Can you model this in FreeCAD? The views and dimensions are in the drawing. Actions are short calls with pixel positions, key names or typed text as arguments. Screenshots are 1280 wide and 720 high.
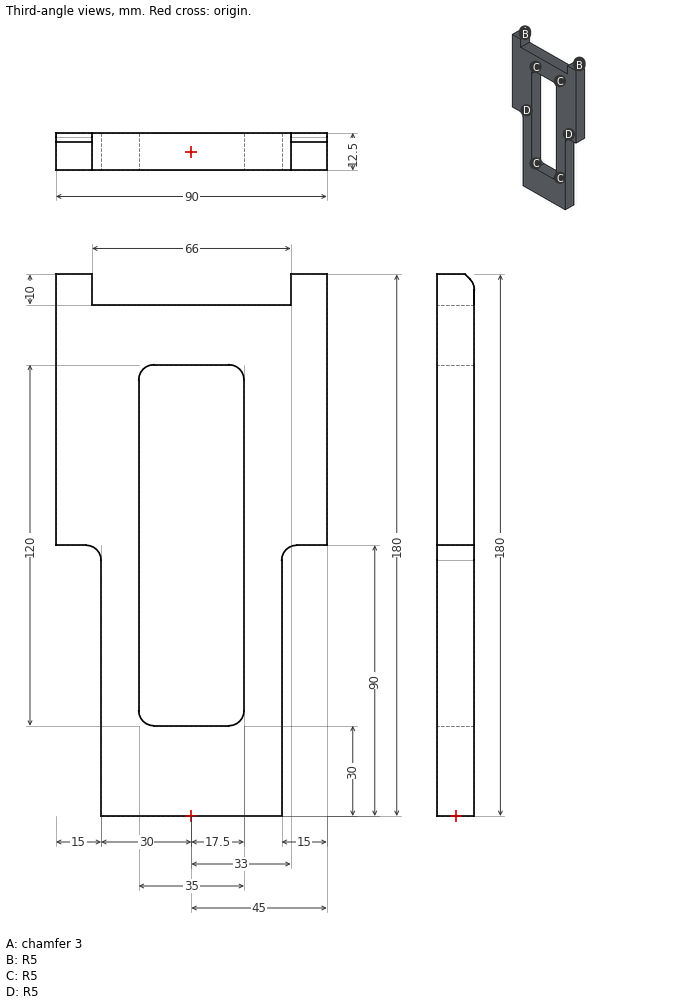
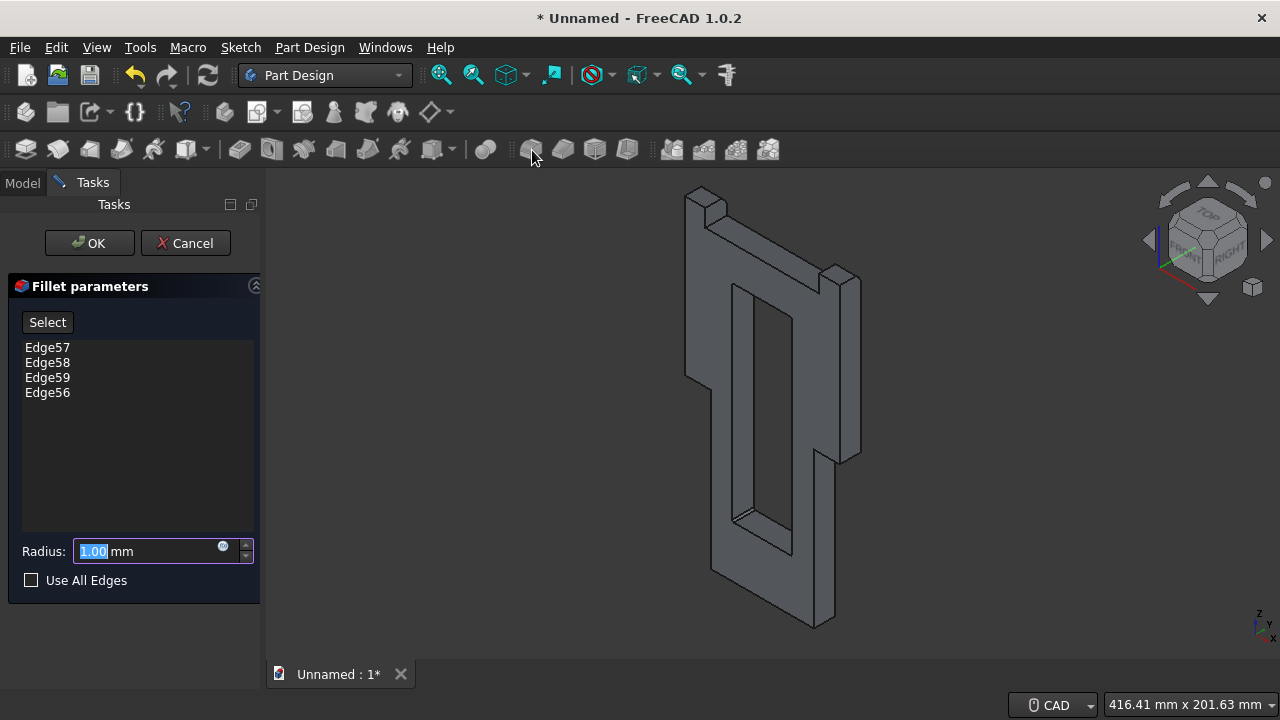
text(5)
key(Tab)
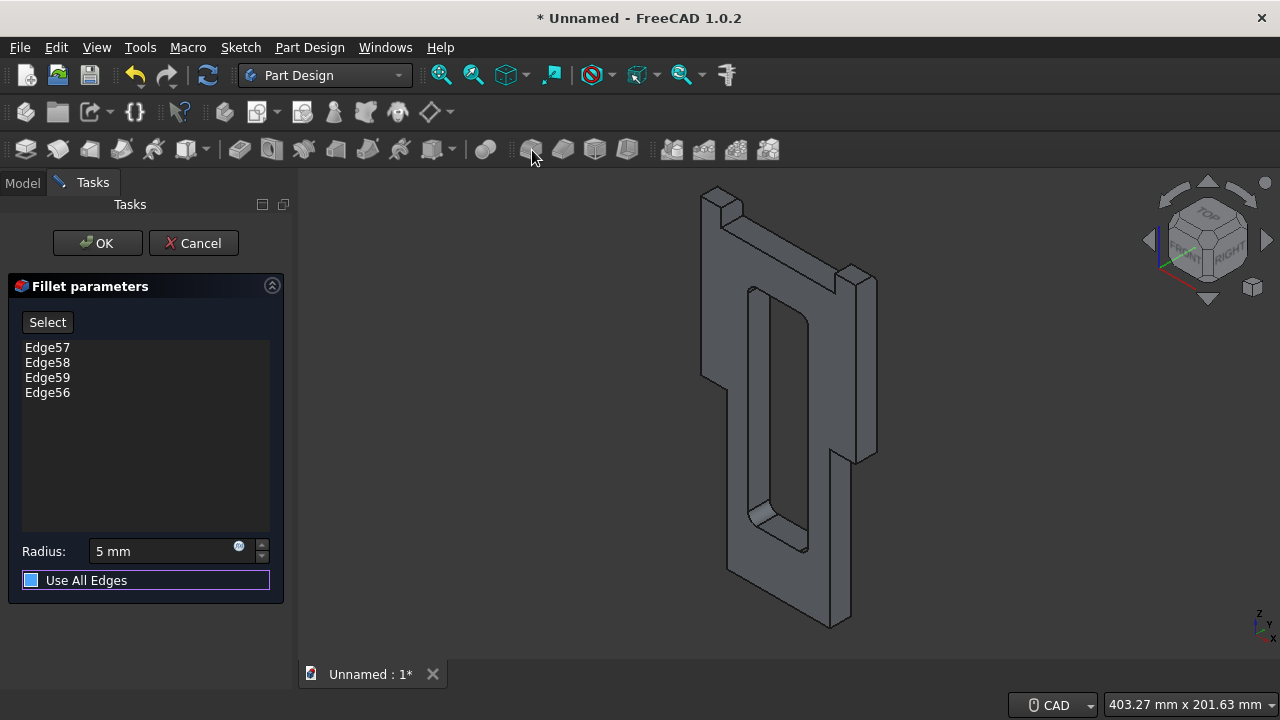
click(98, 243)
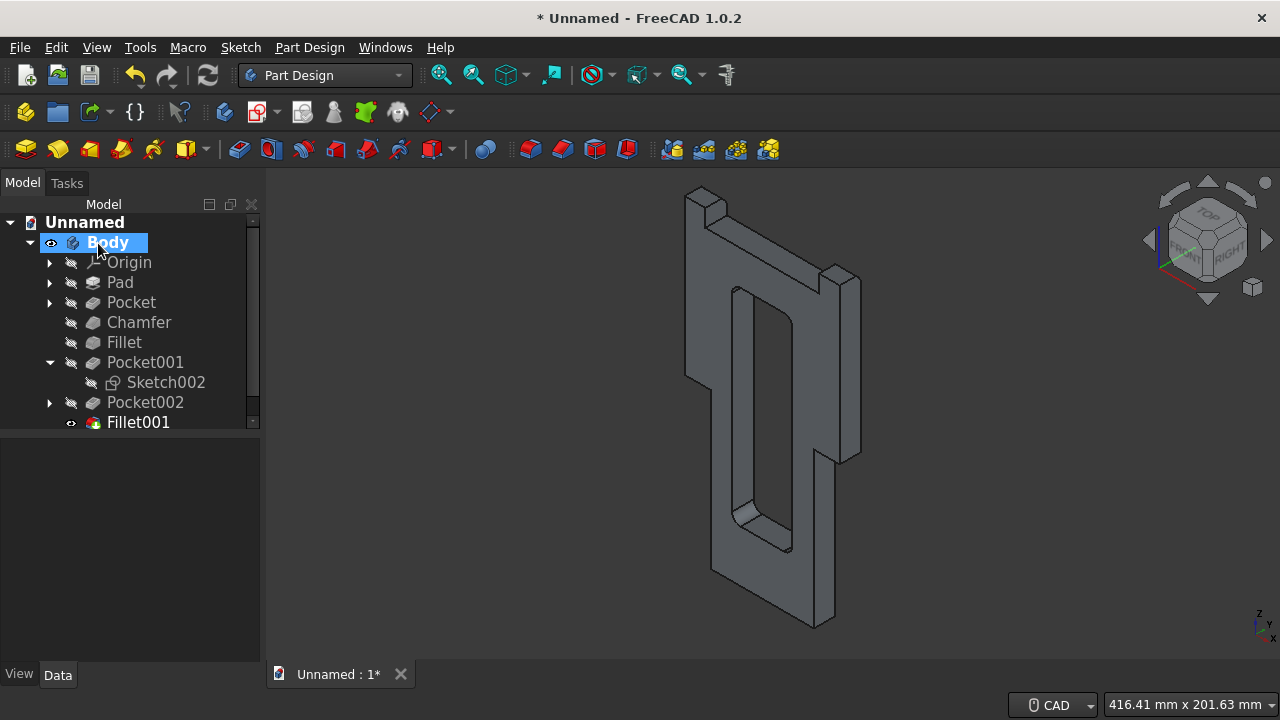
key(2)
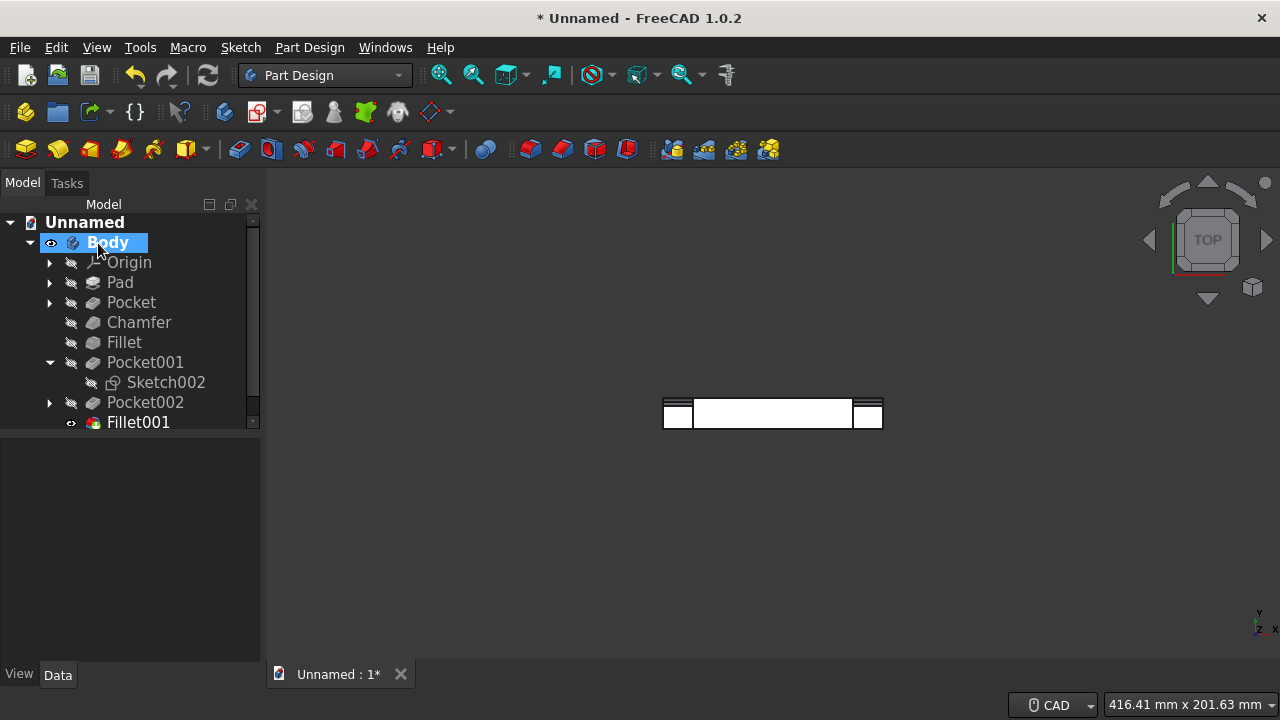
click(442, 76)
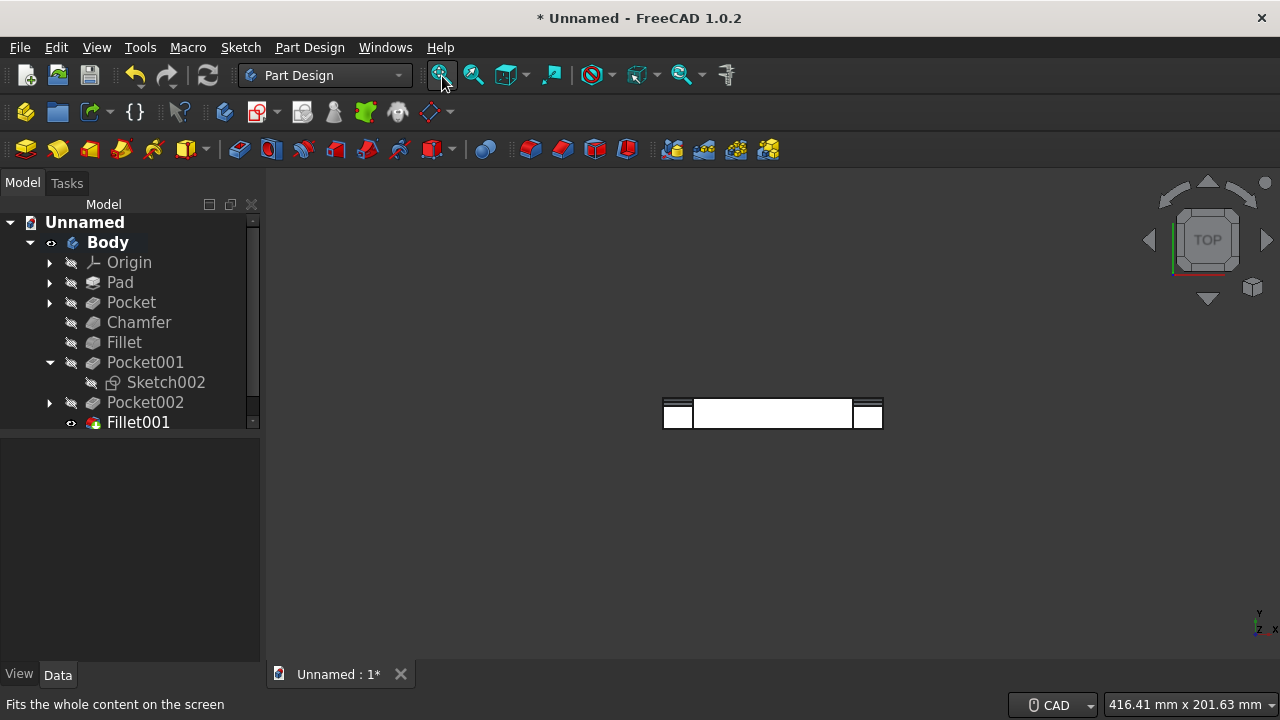
key(0)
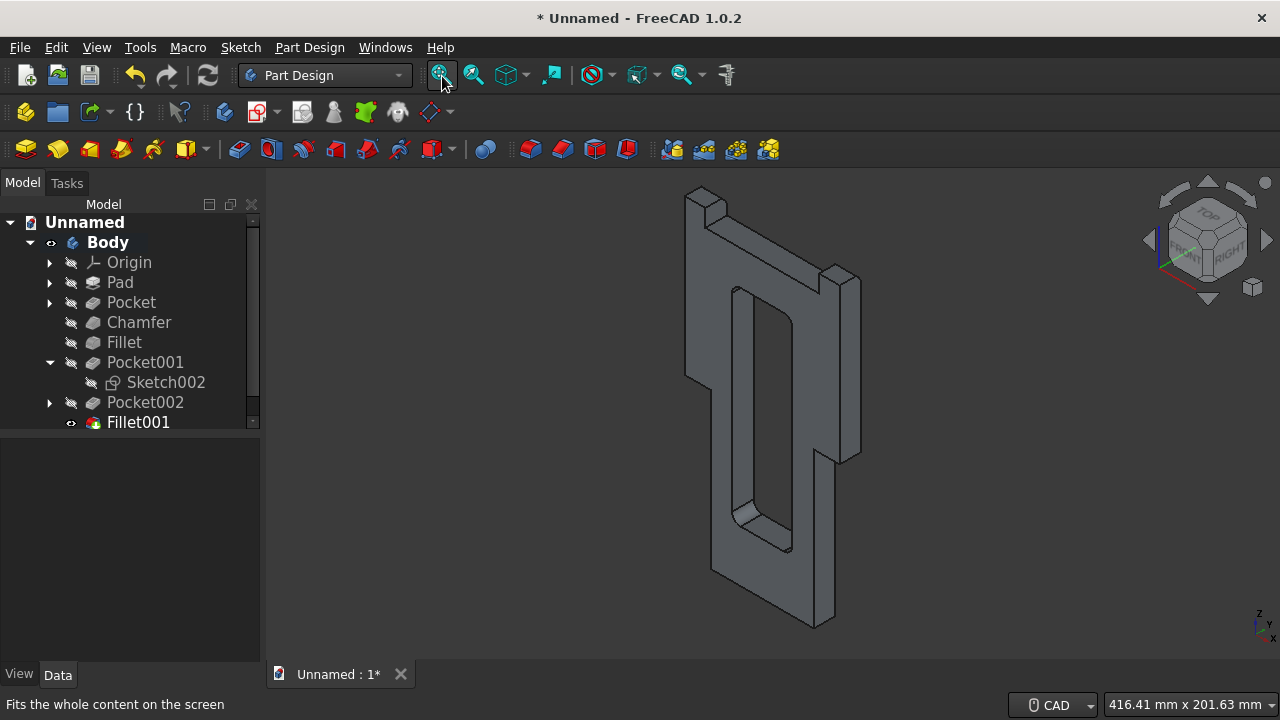
key(1)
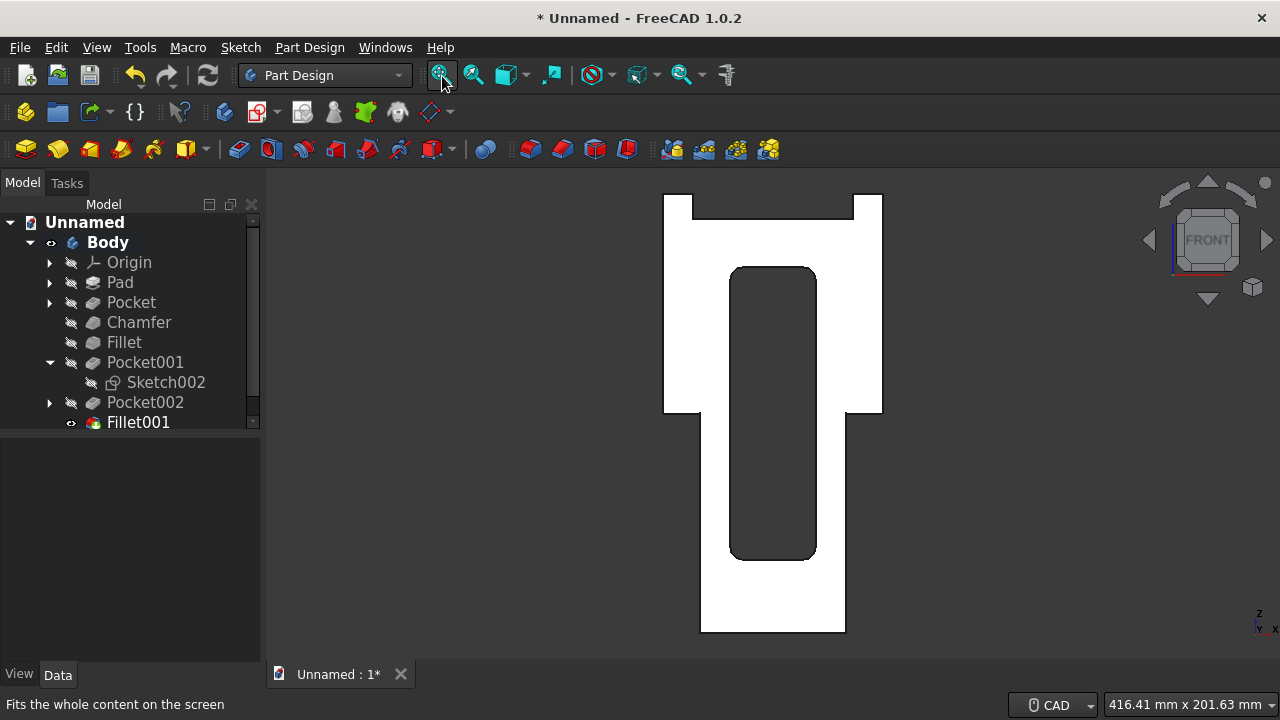
key(3)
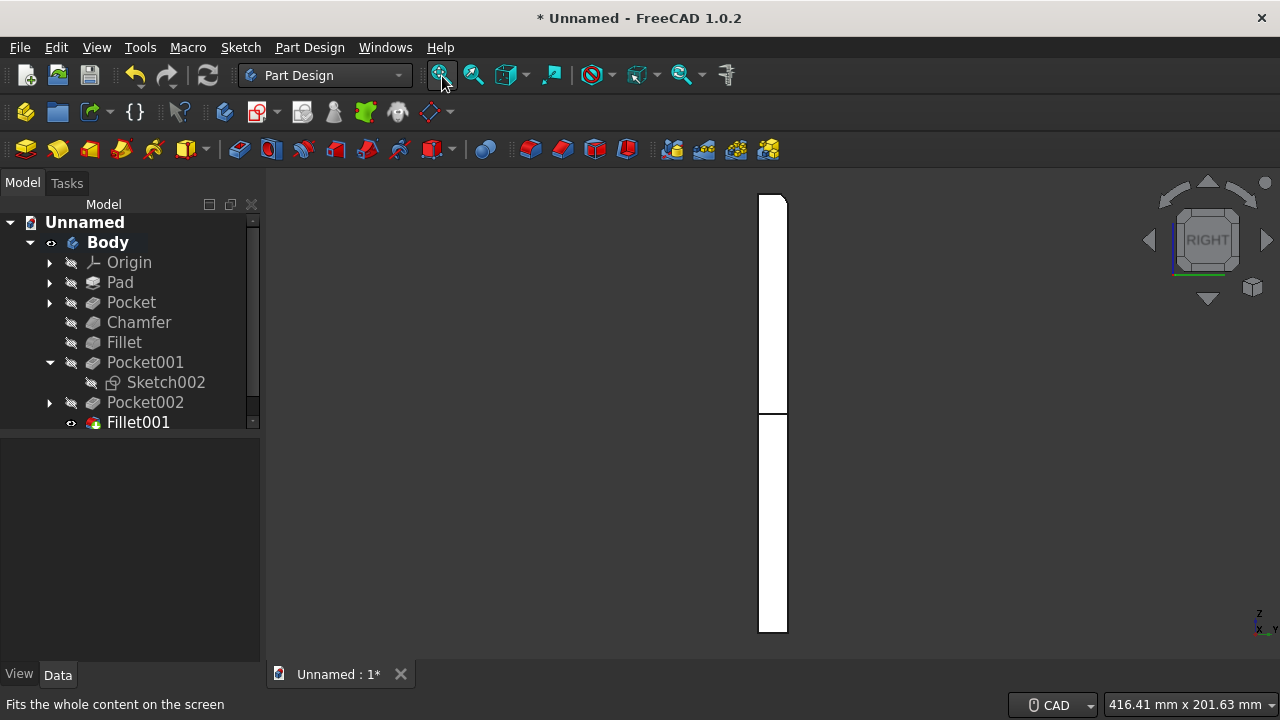
key(5)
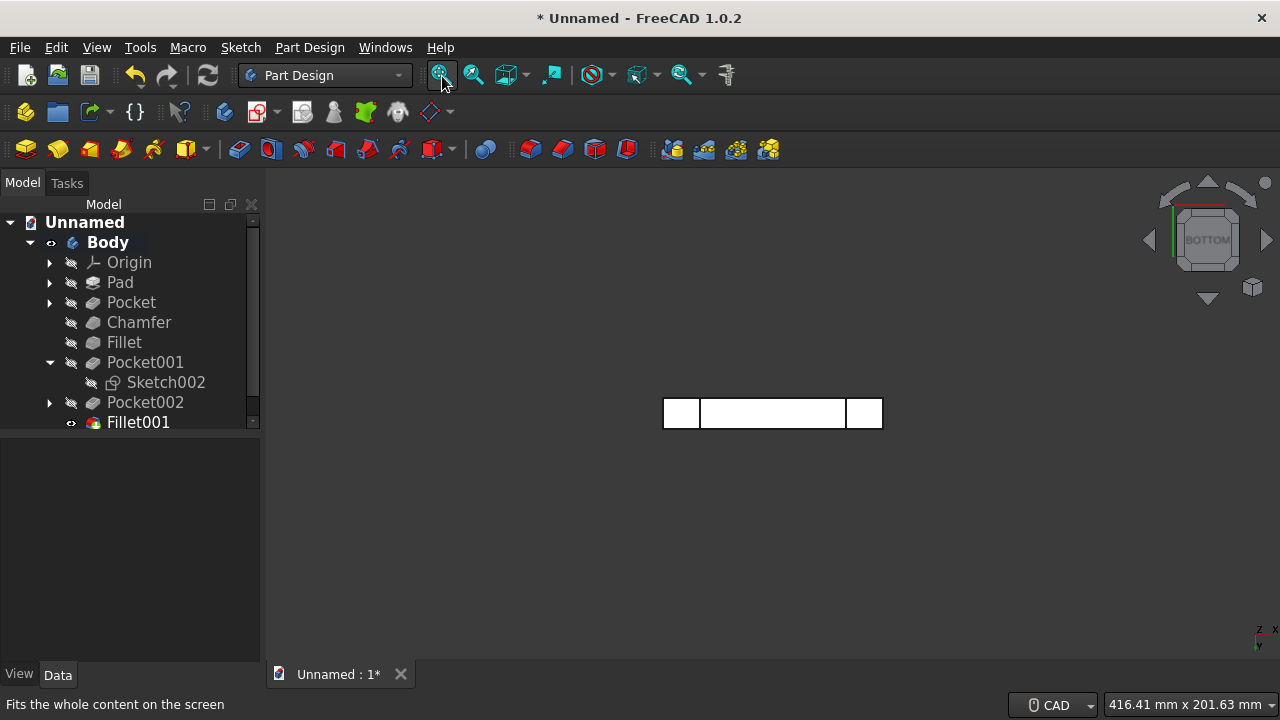
click(442, 76)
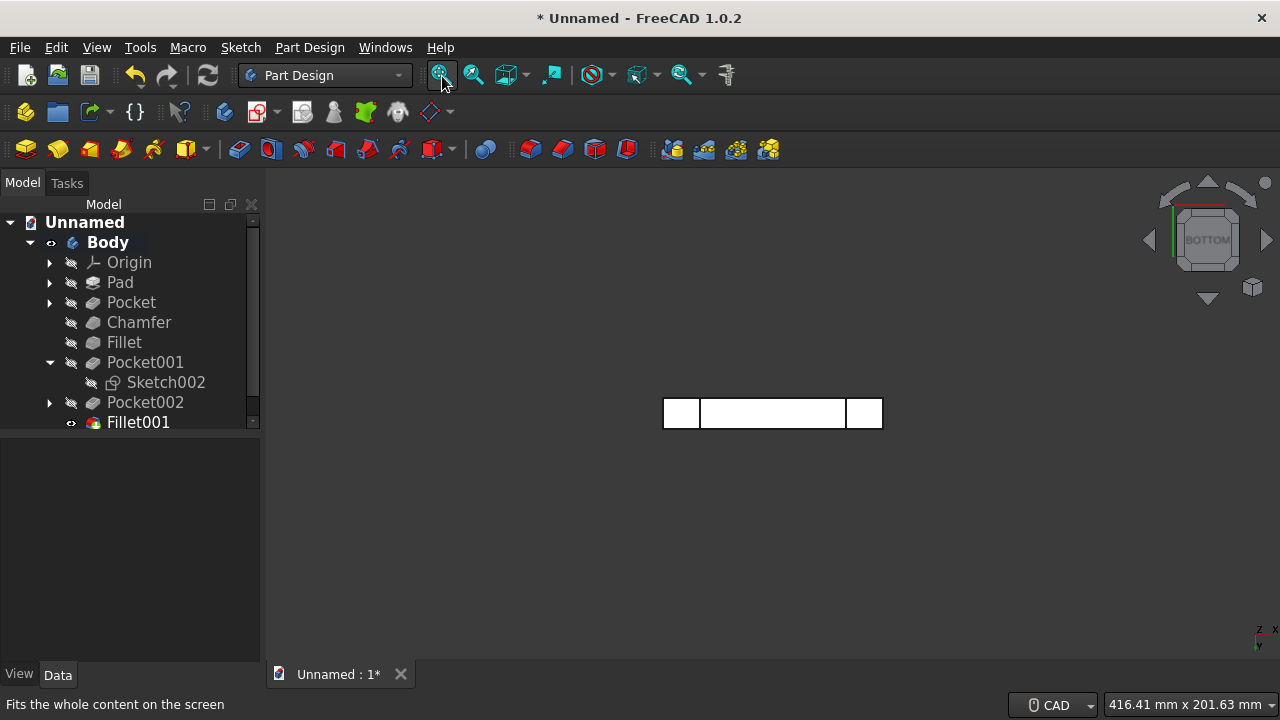
key(4)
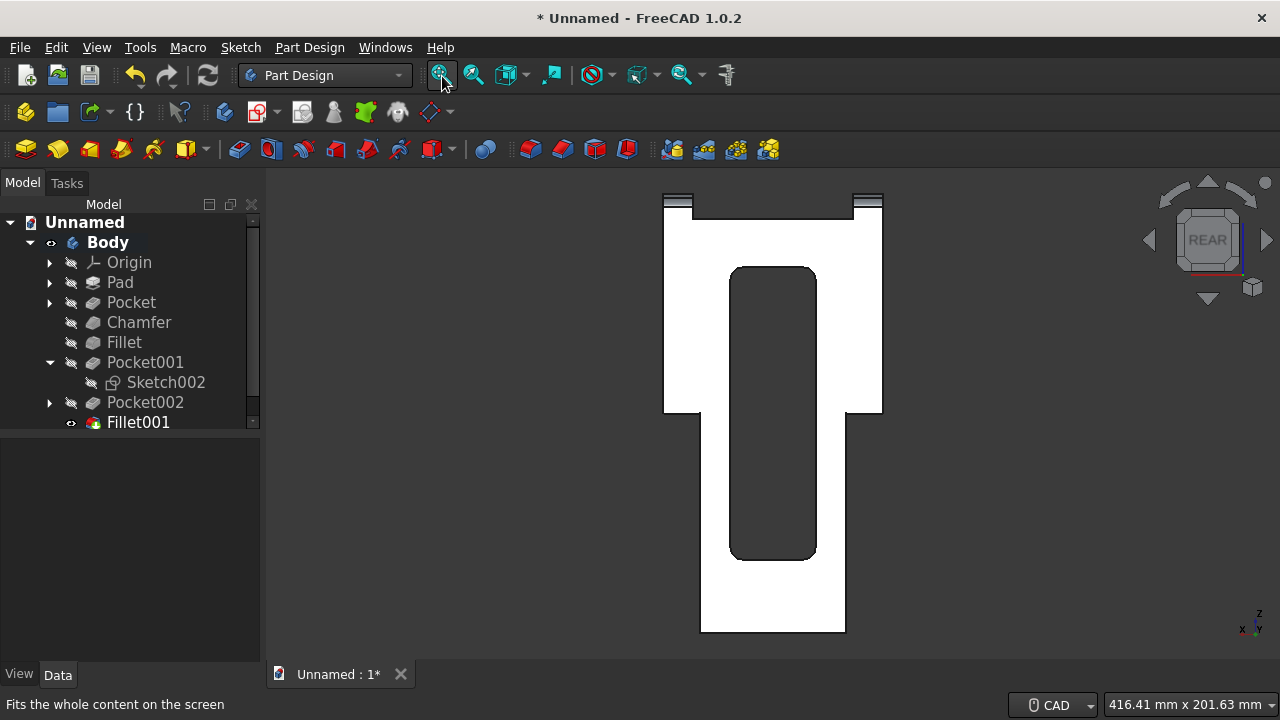
key(6)